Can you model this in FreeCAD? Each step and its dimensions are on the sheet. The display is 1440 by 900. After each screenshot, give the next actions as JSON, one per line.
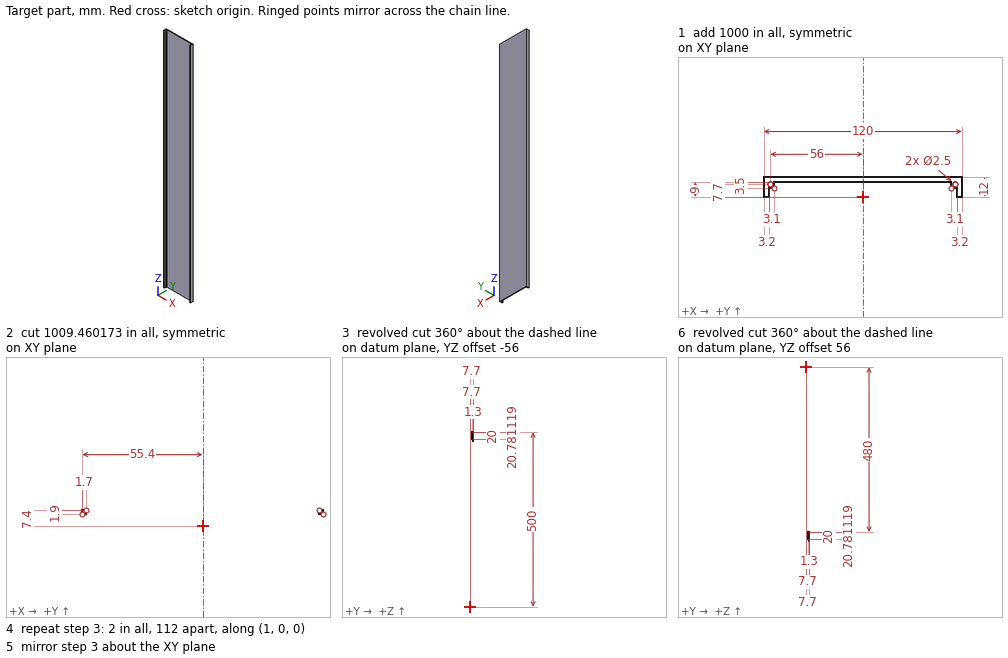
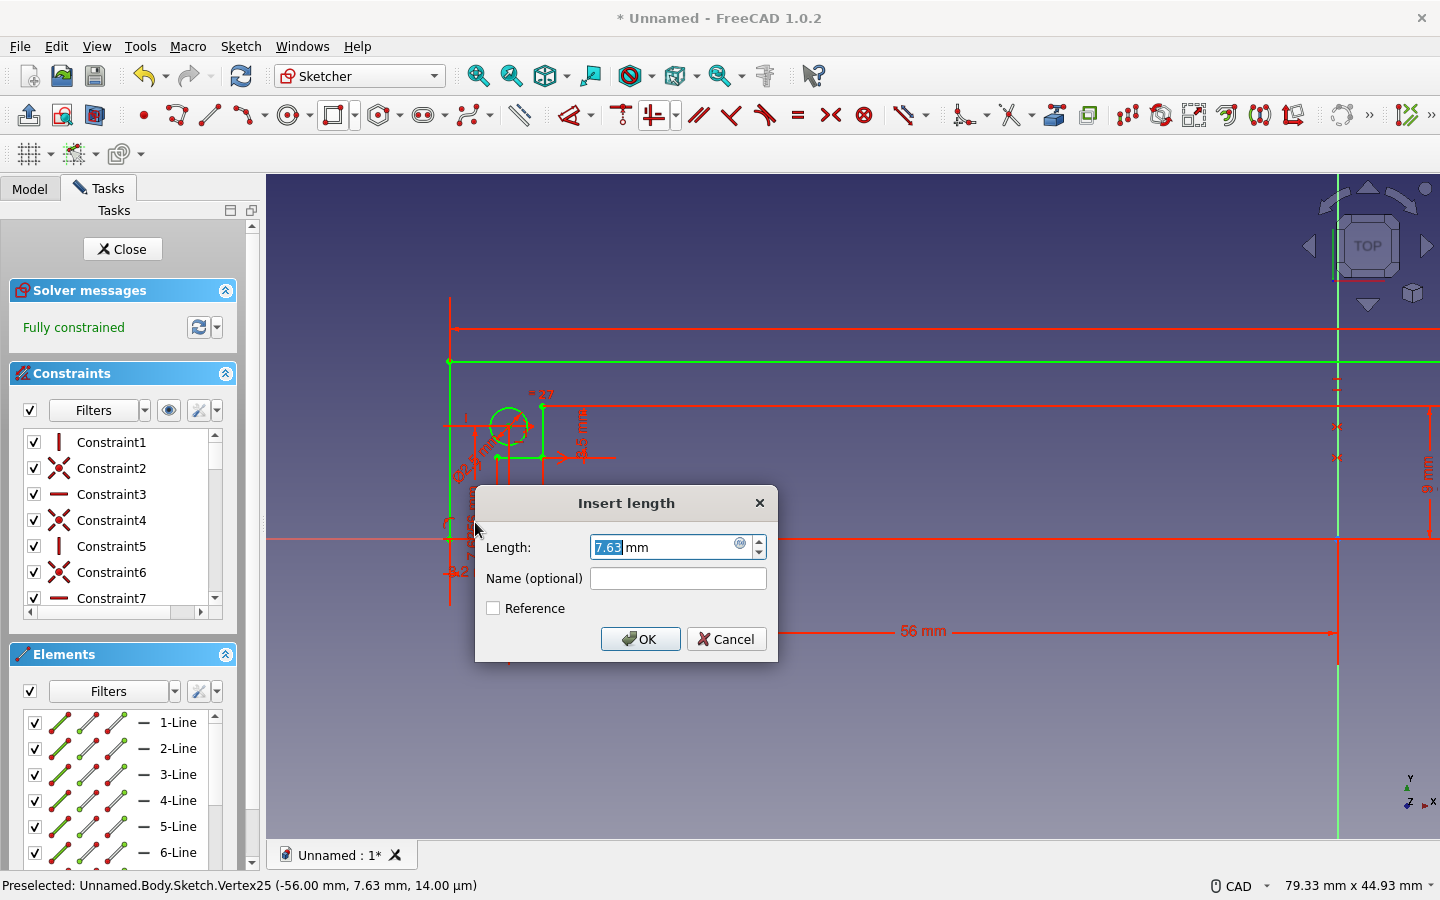
{"action": "type", "text": "7.7"}
{"action": "key", "text": "Return"}
{"action": "key", "text": "Escape"}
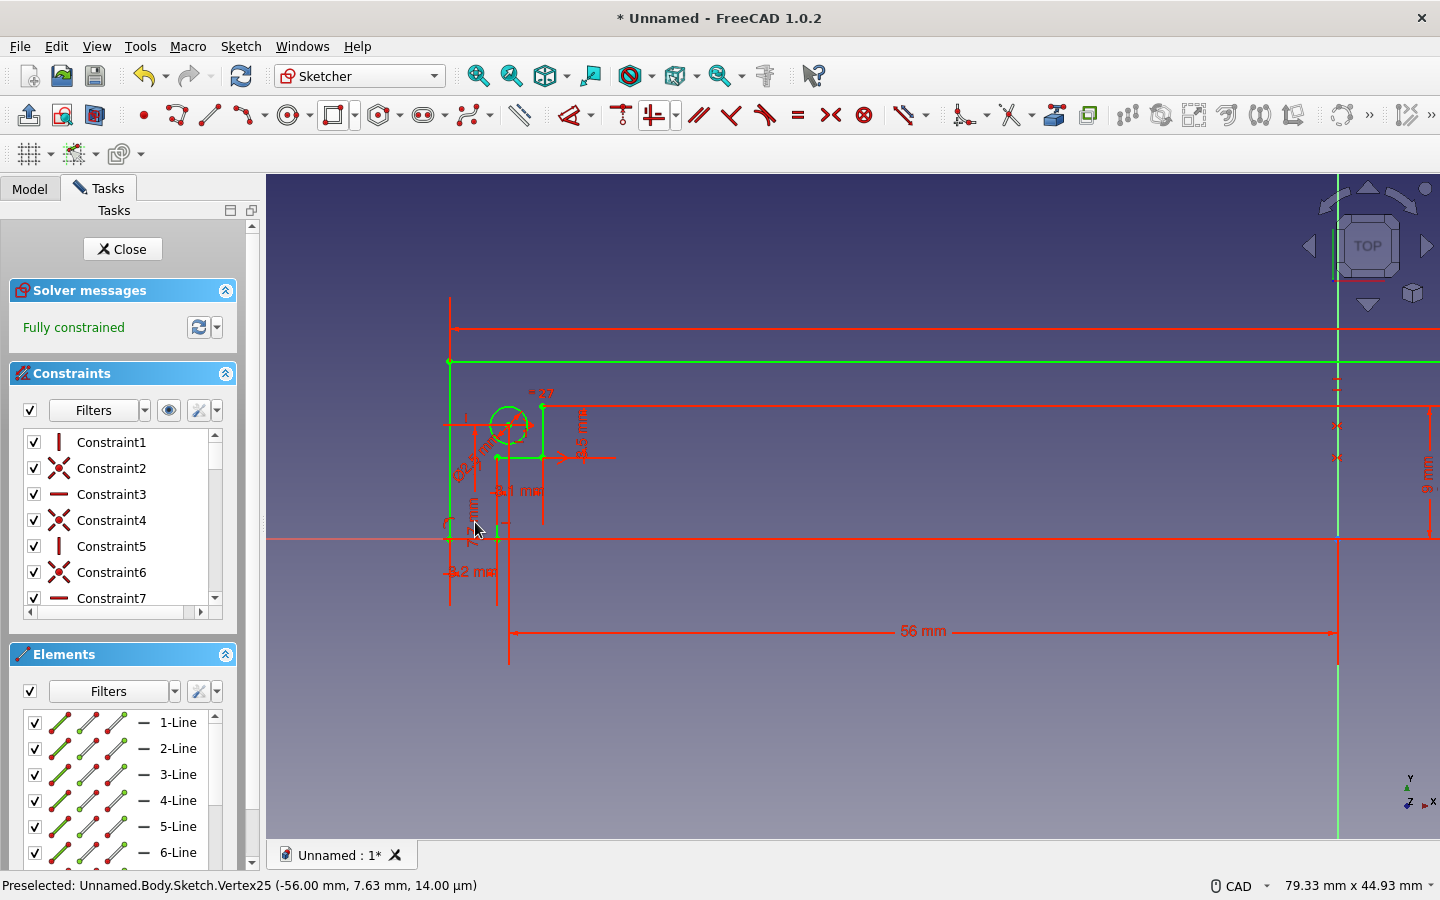
{"action": "left_click", "coordinate": [123, 249]}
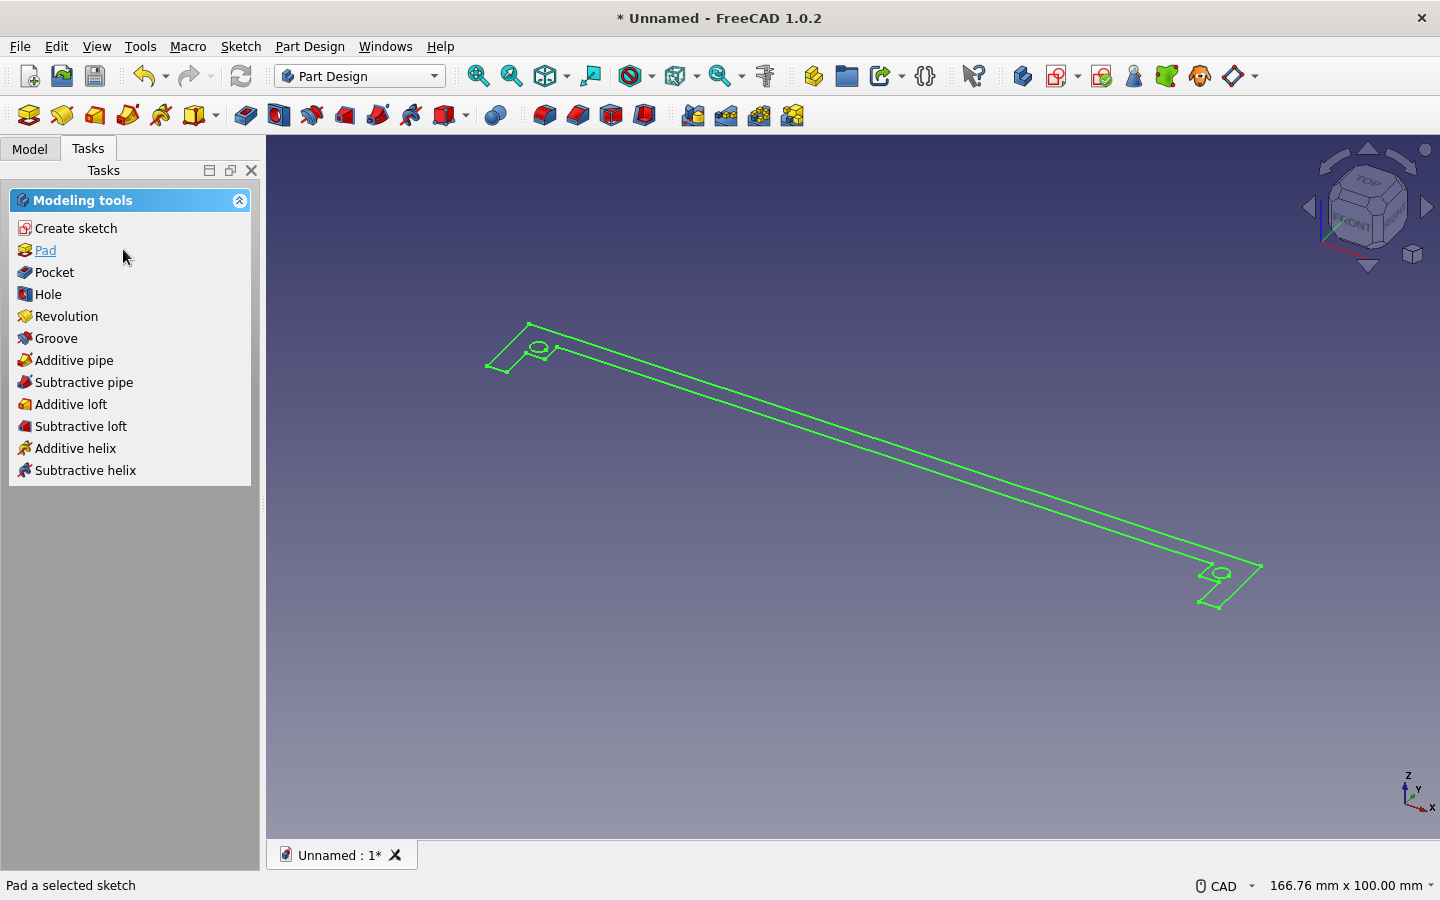
{"action": "left_click", "coordinate": [29, 116]}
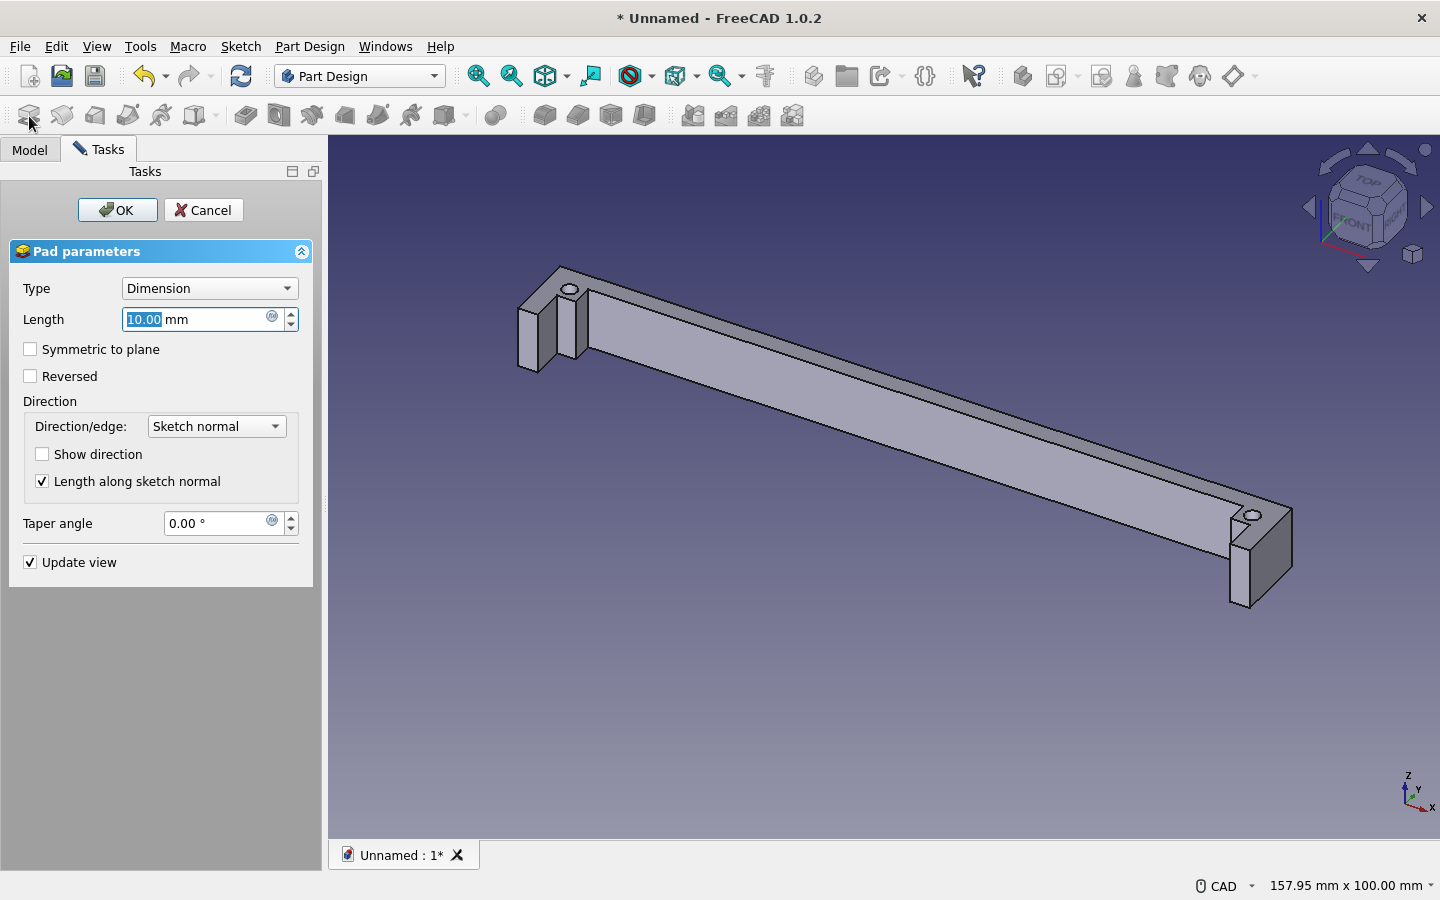
{"action": "type", "text": "1000"}
{"action": "key", "text": "Tab"}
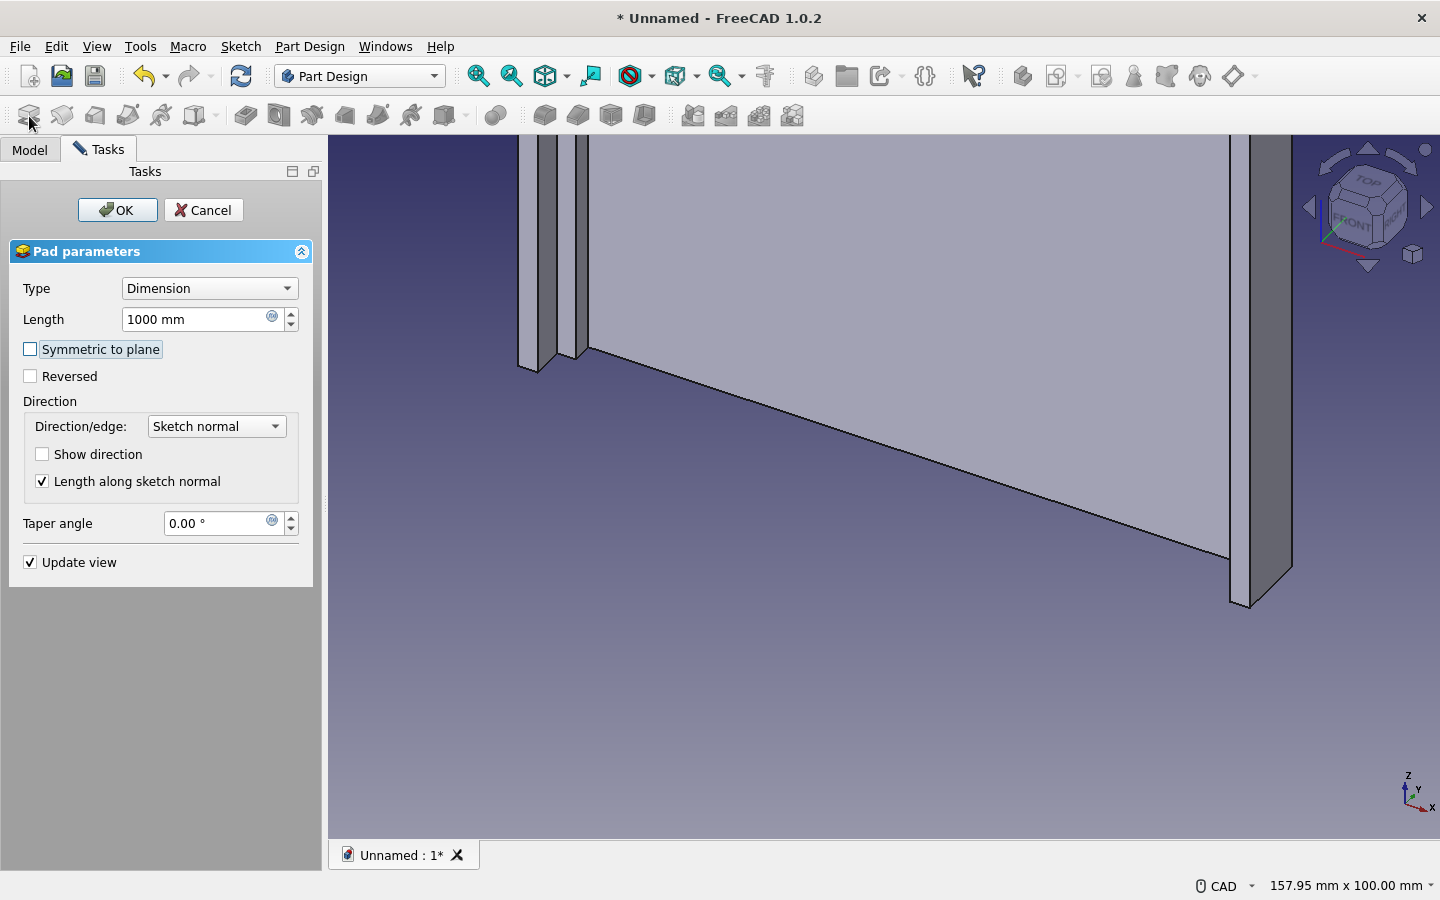
{"action": "left_click", "coordinate": [31, 349]}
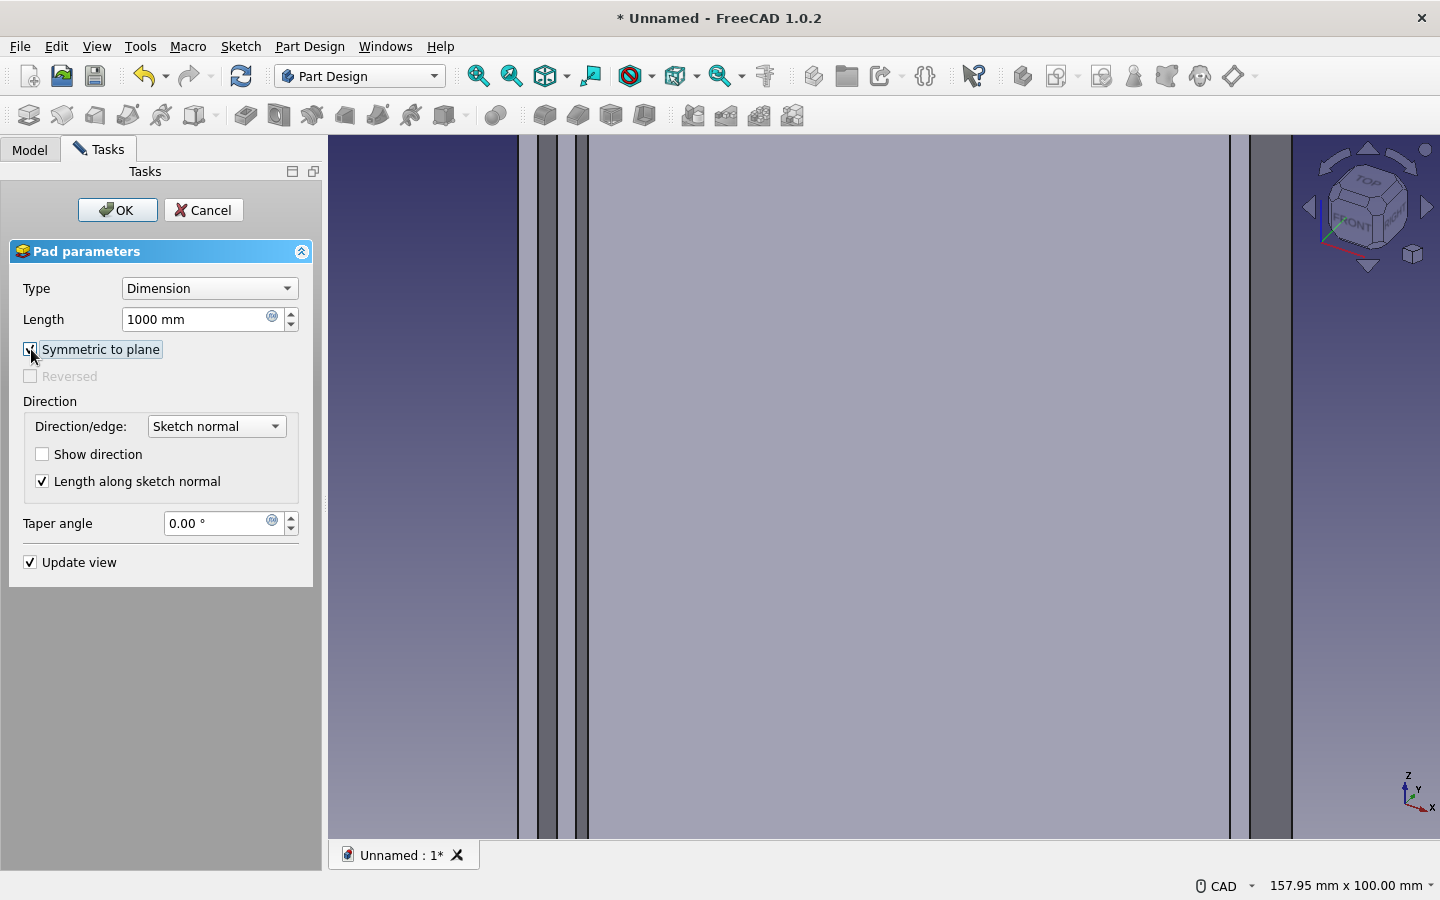
{"action": "left_click", "coordinate": [118, 210]}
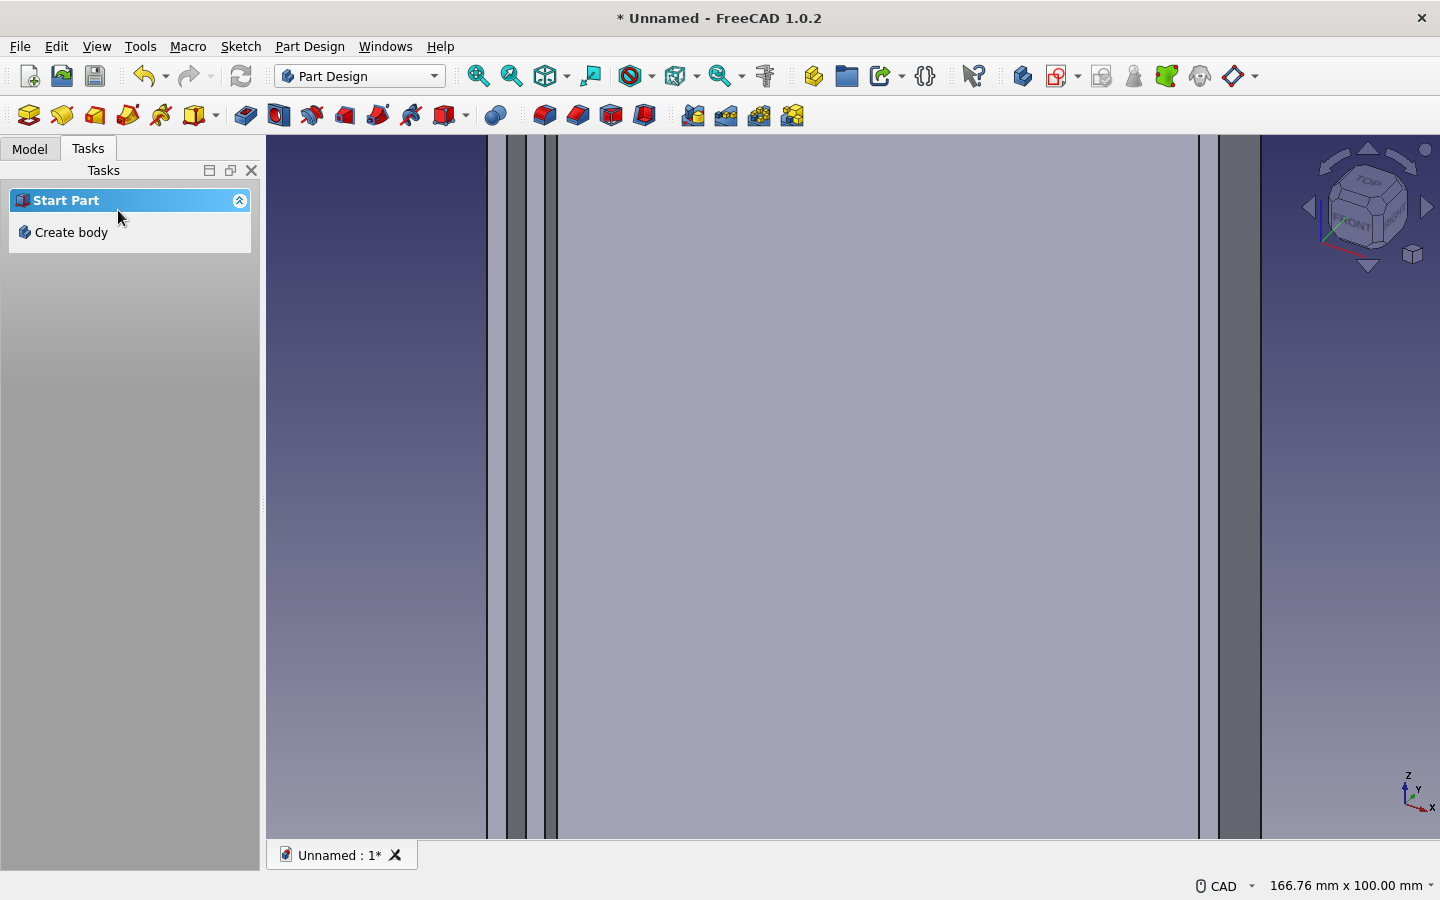
{"action": "left_click", "coordinate": [479, 76]}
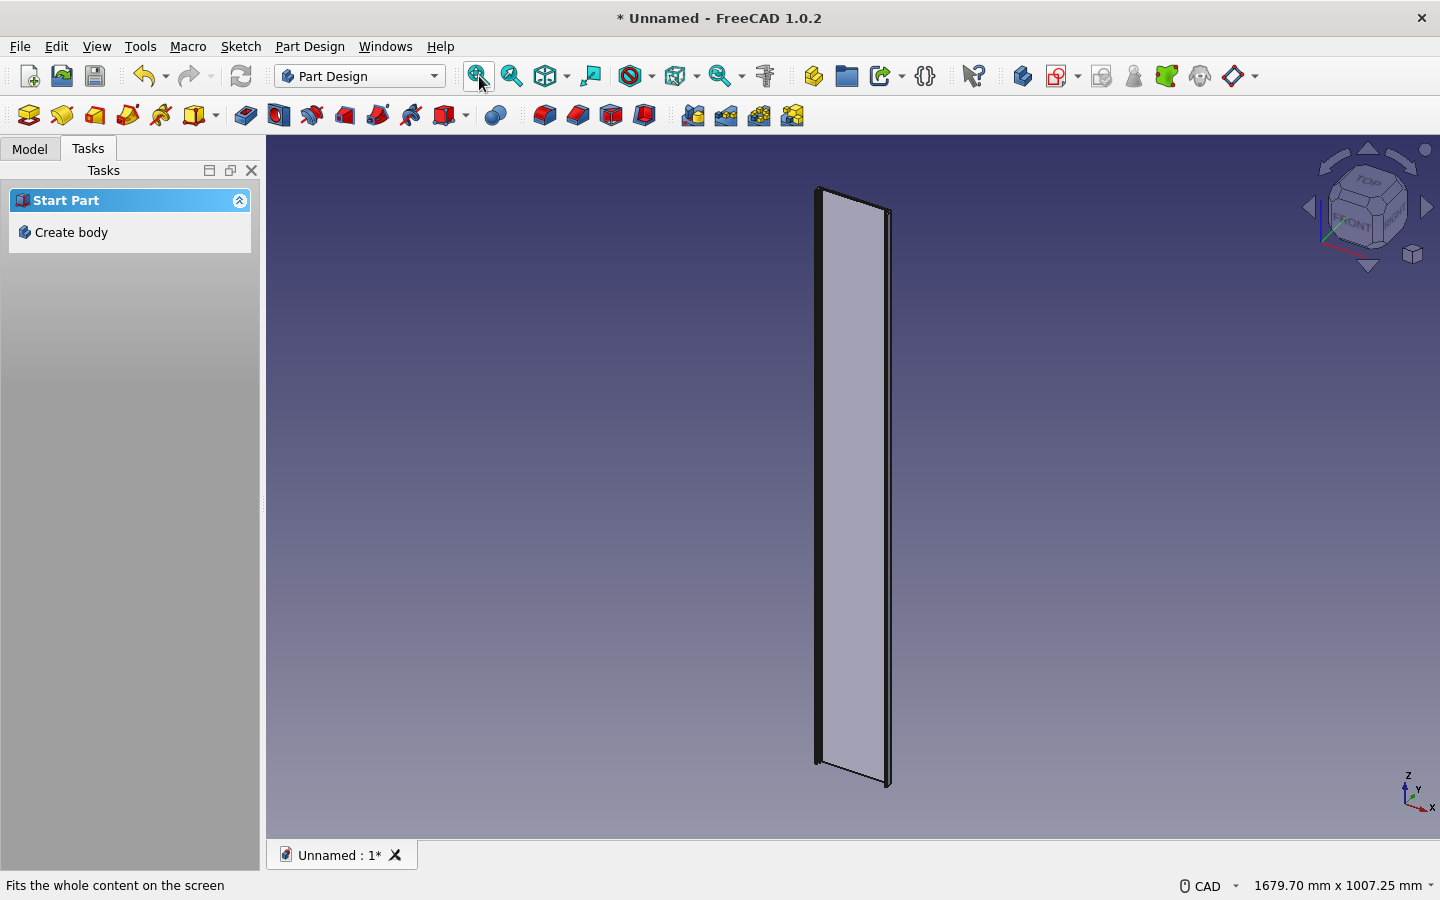
{"action": "left_click", "coordinate": [1056, 76]}